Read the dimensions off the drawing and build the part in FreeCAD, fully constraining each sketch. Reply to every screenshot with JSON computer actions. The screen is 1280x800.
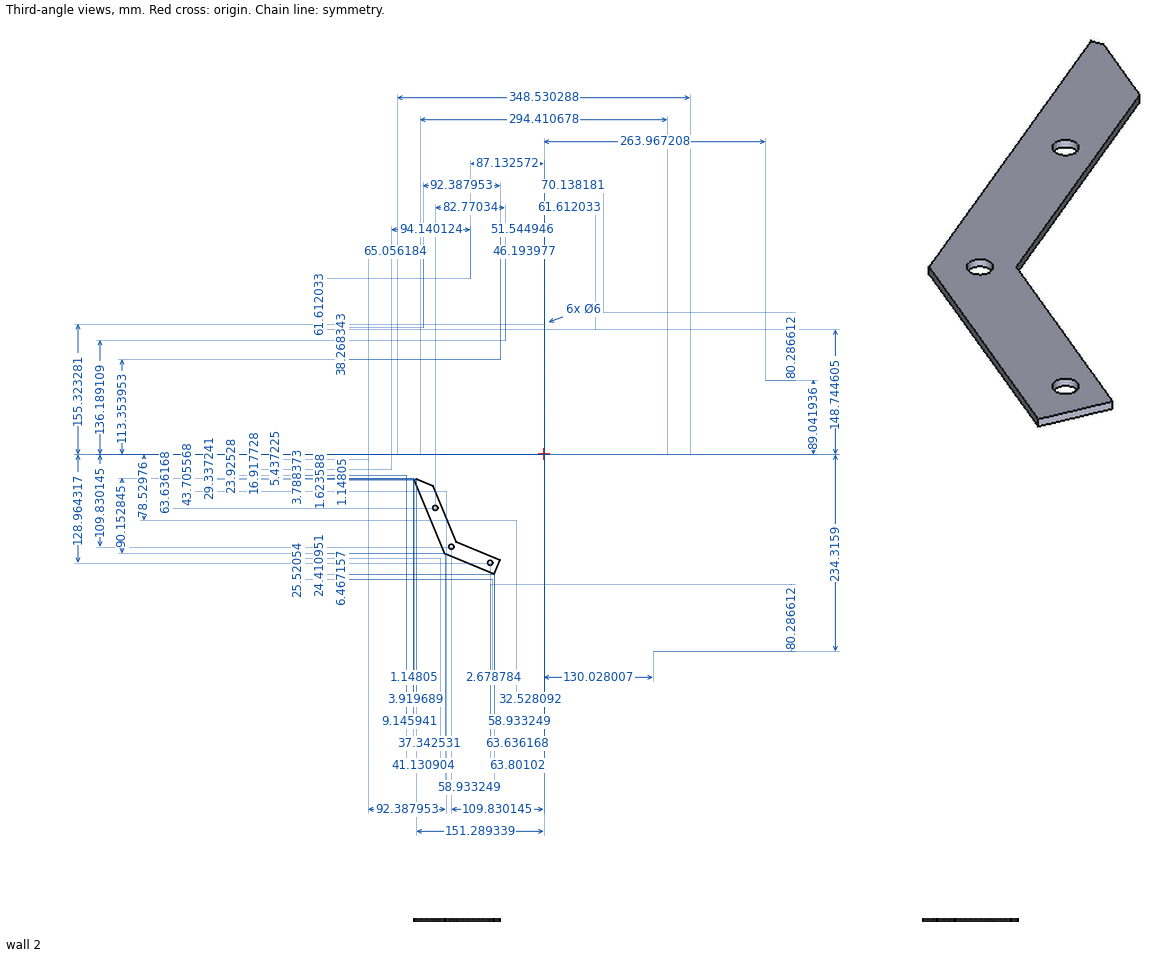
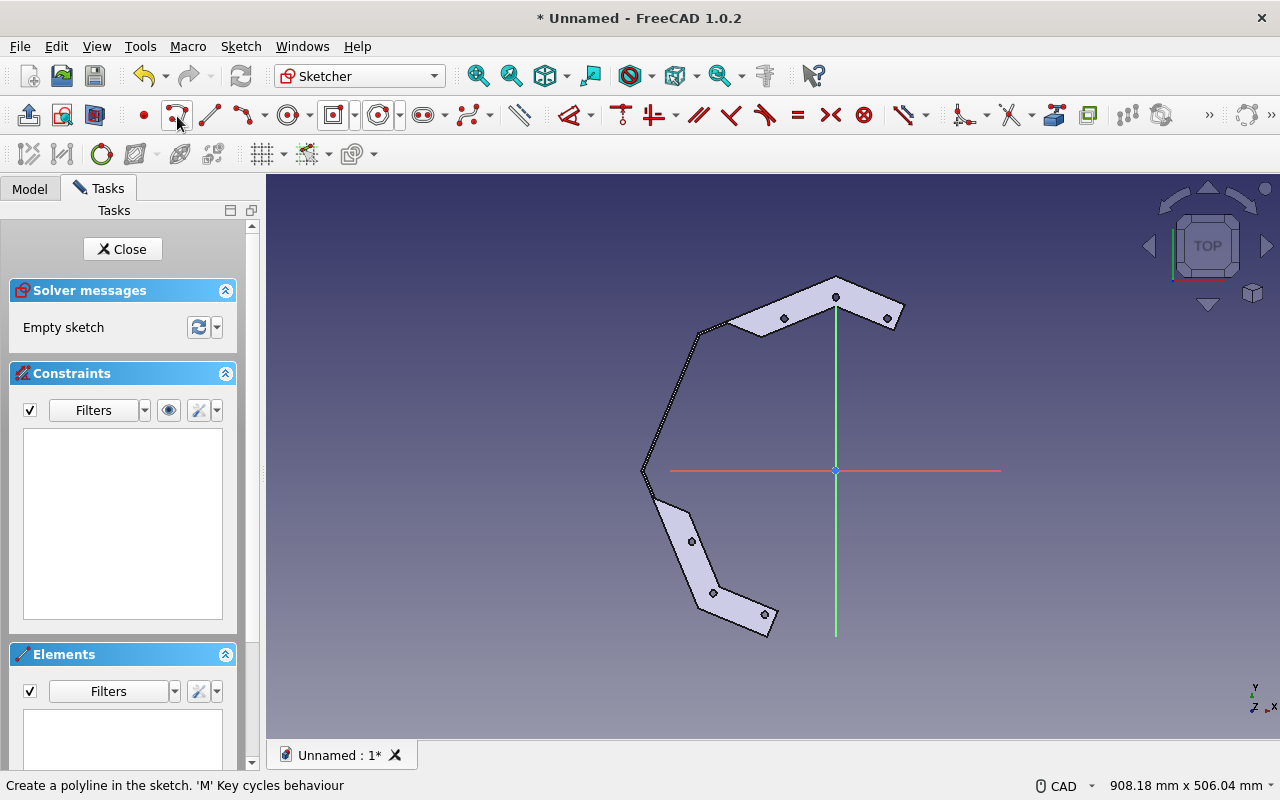
{"action": "left_click", "coordinate": [800, 558]}
{"action": "left_click", "coordinate": [905, 305]}
{"action": "left_click", "coordinate": [739, 236]}
{"action": "left_click", "coordinate": [633, 490]}
{"action": "left_click", "coordinate": [800, 559]}
{"action": "key", "text": "Escape"}
{"action": "key", "text": "Escape"}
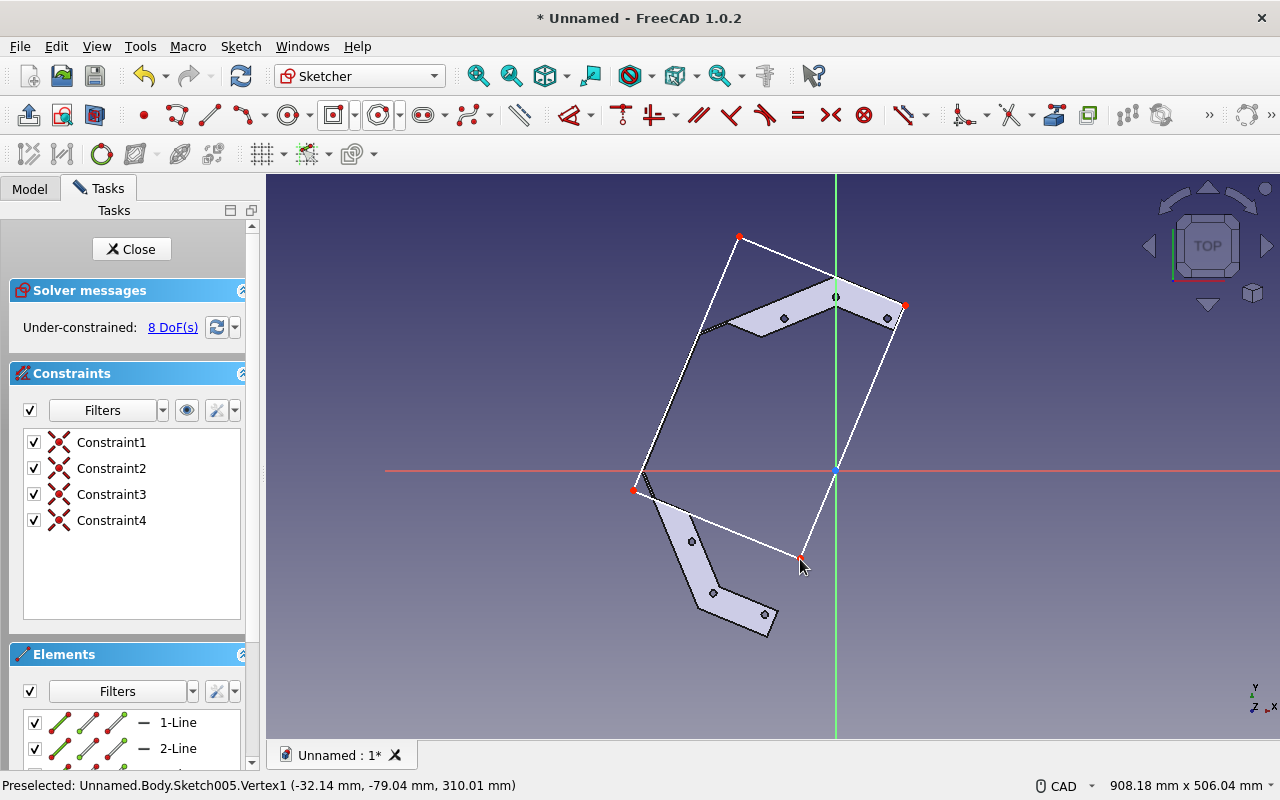
{"action": "left_click", "coordinate": [568, 116]}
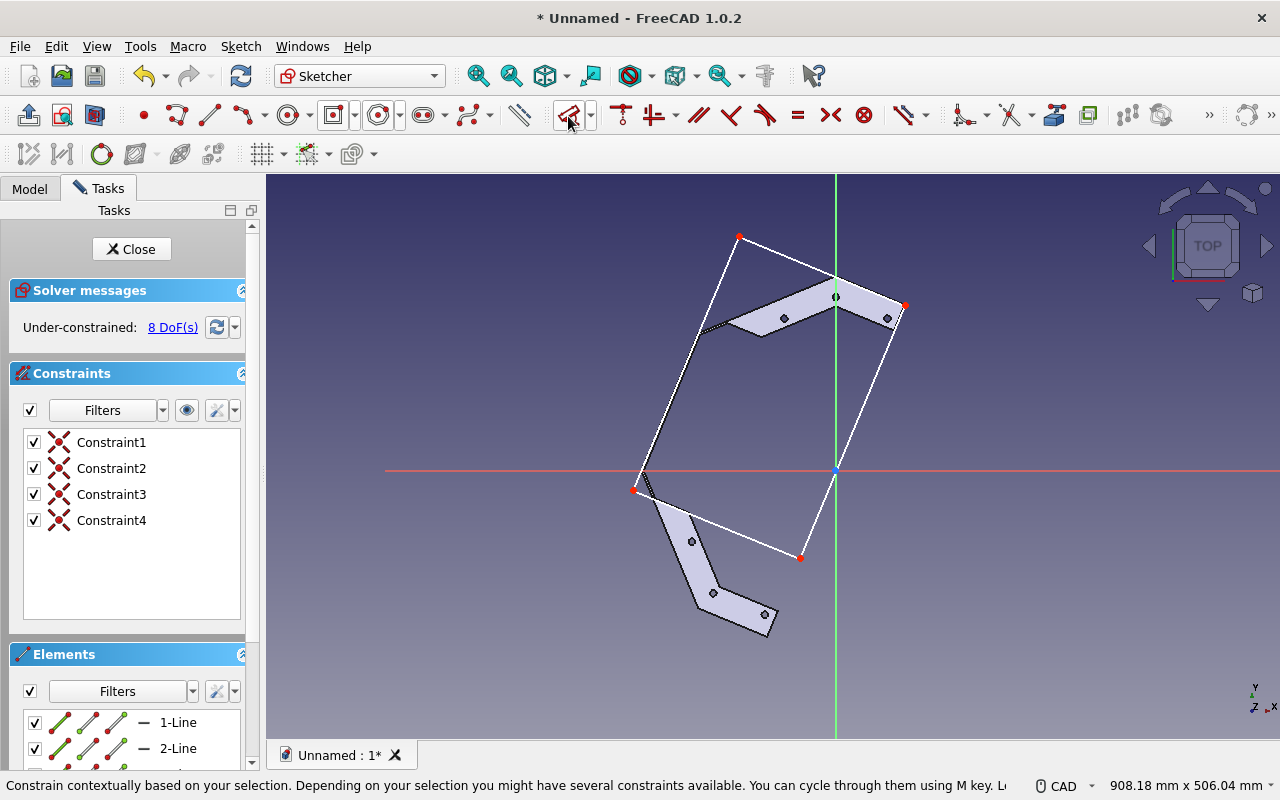
{"action": "left_click", "coordinate": [800, 559]}
{"action": "left_click", "coordinate": [870, 515]}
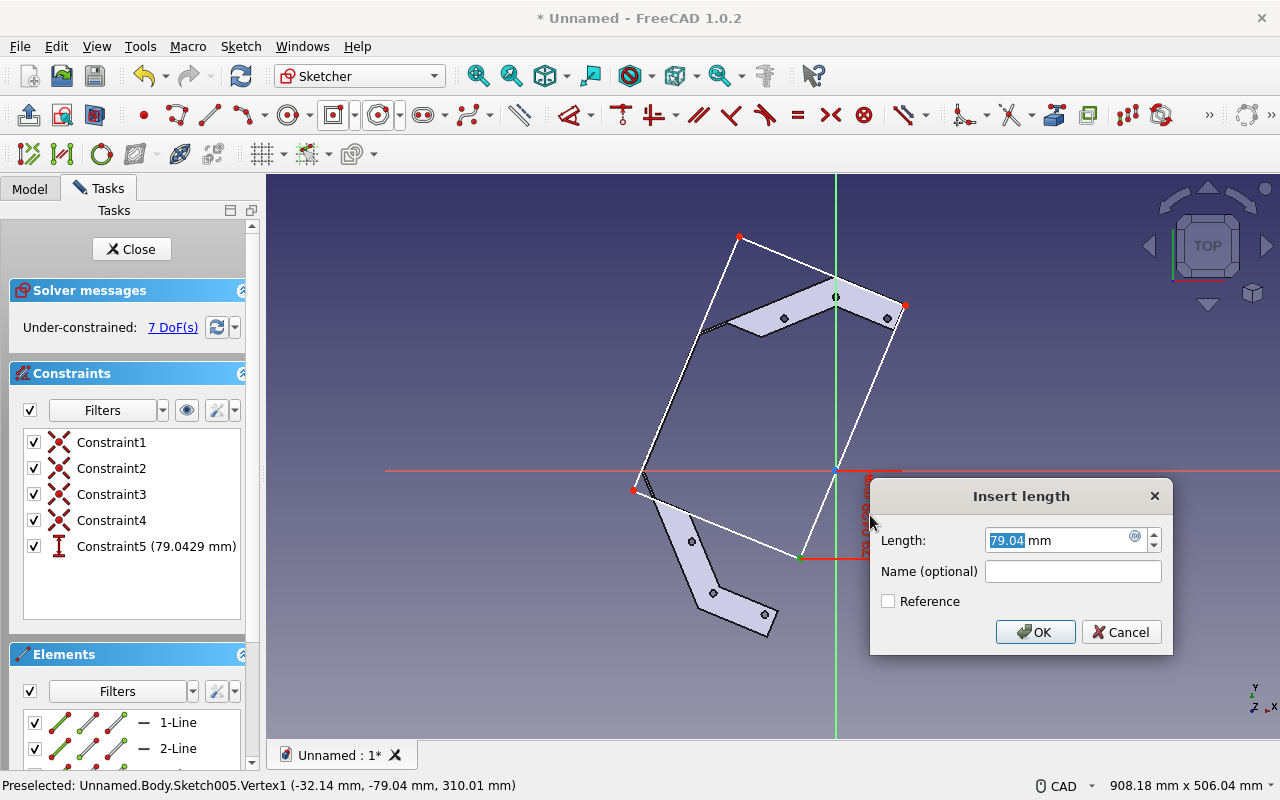
{"action": "type", "text": "78.52976"}
{"action": "key", "text": "Return"}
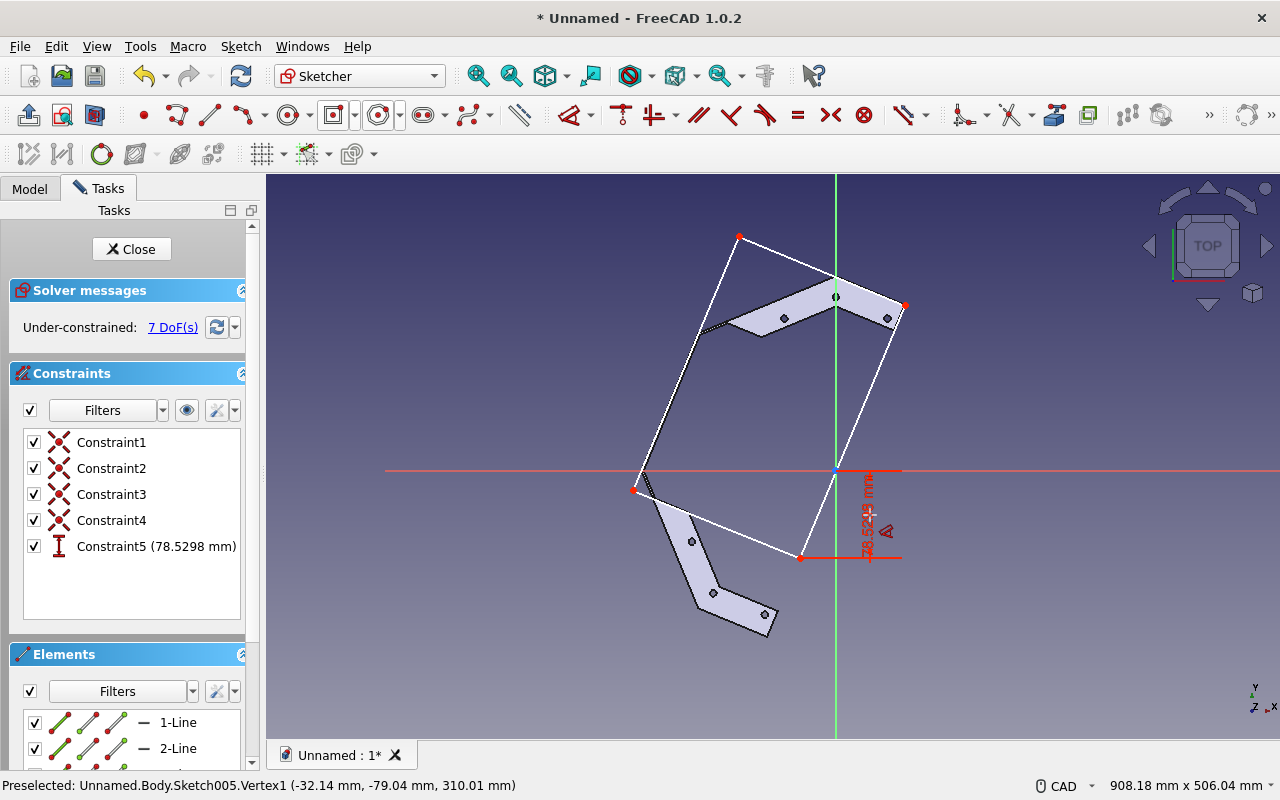
{"action": "left_click", "coordinate": [800, 558]}
{"action": "left_click", "coordinate": [818, 592]}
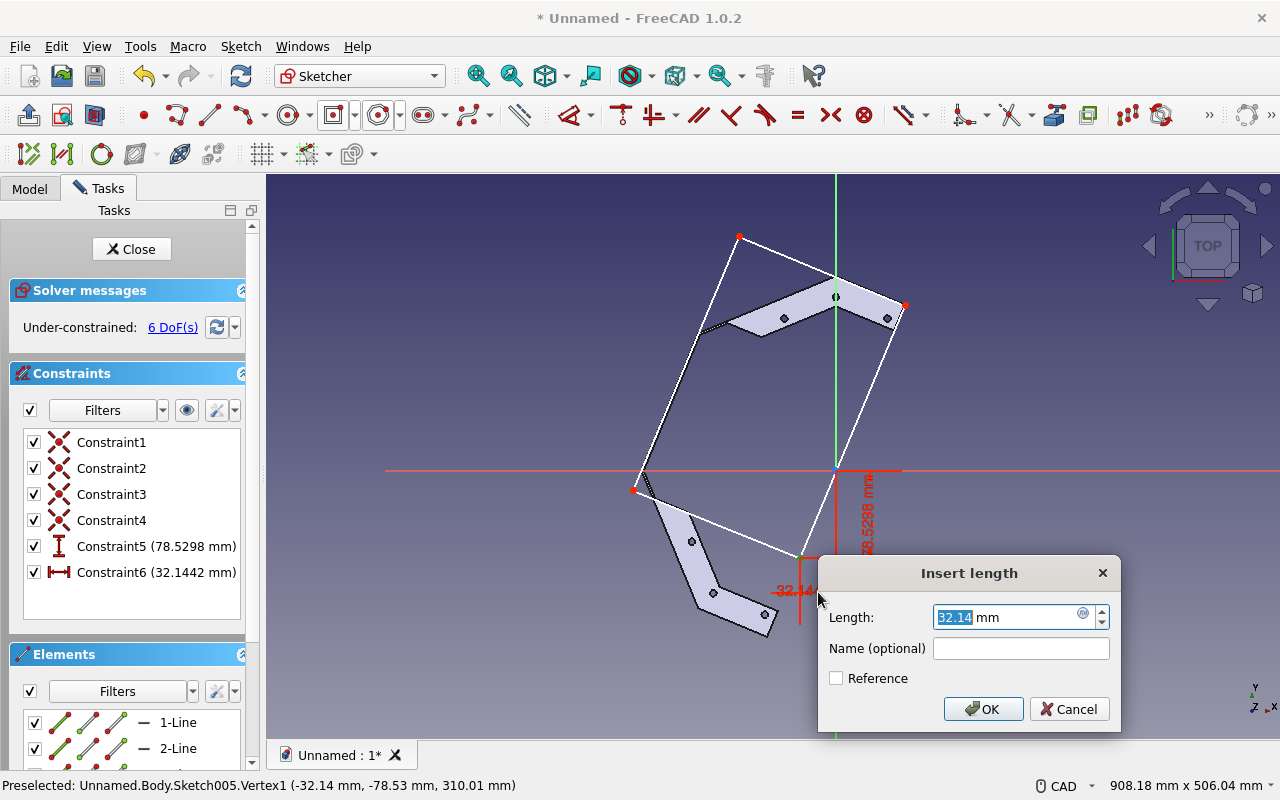
{"action": "type", "text": "32.528092"}
{"action": "key", "text": "Return"}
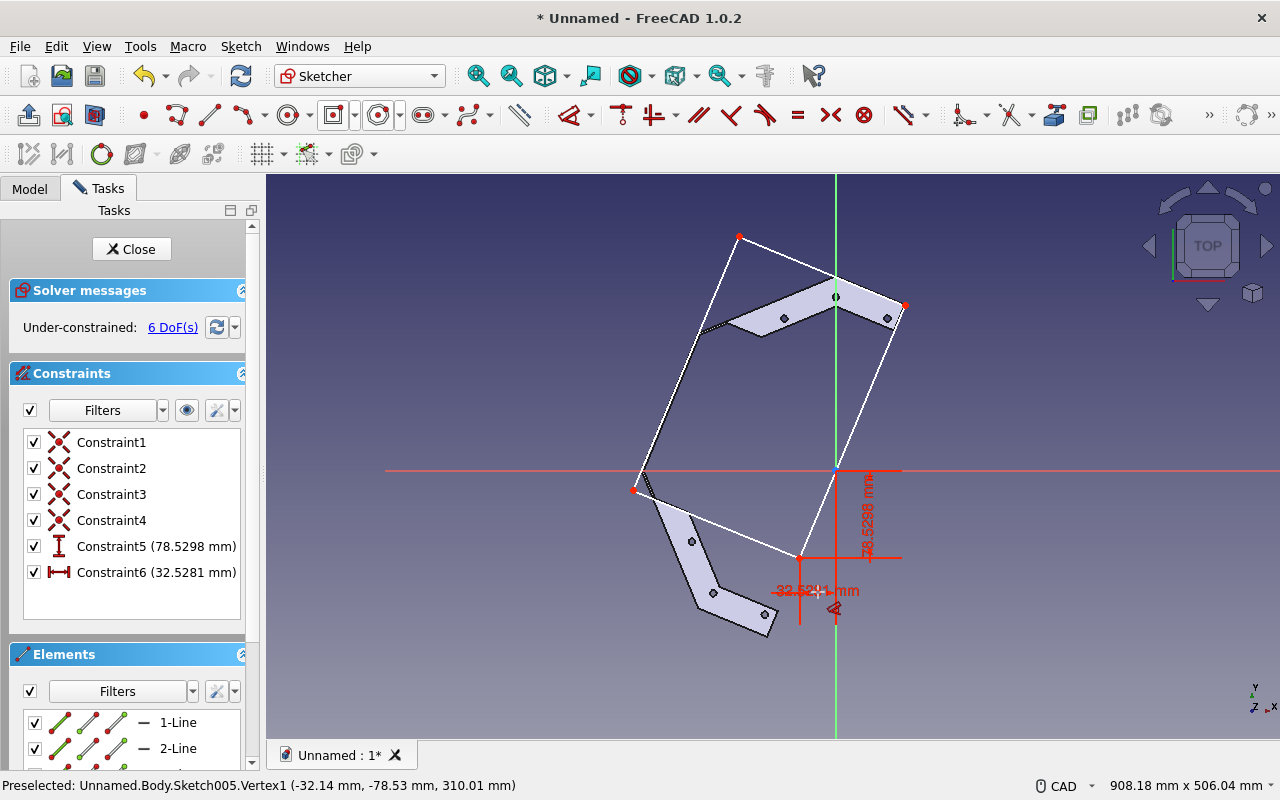
{"action": "left_click", "coordinate": [905, 306]}
{"action": "left_click", "coordinate": [870, 272]}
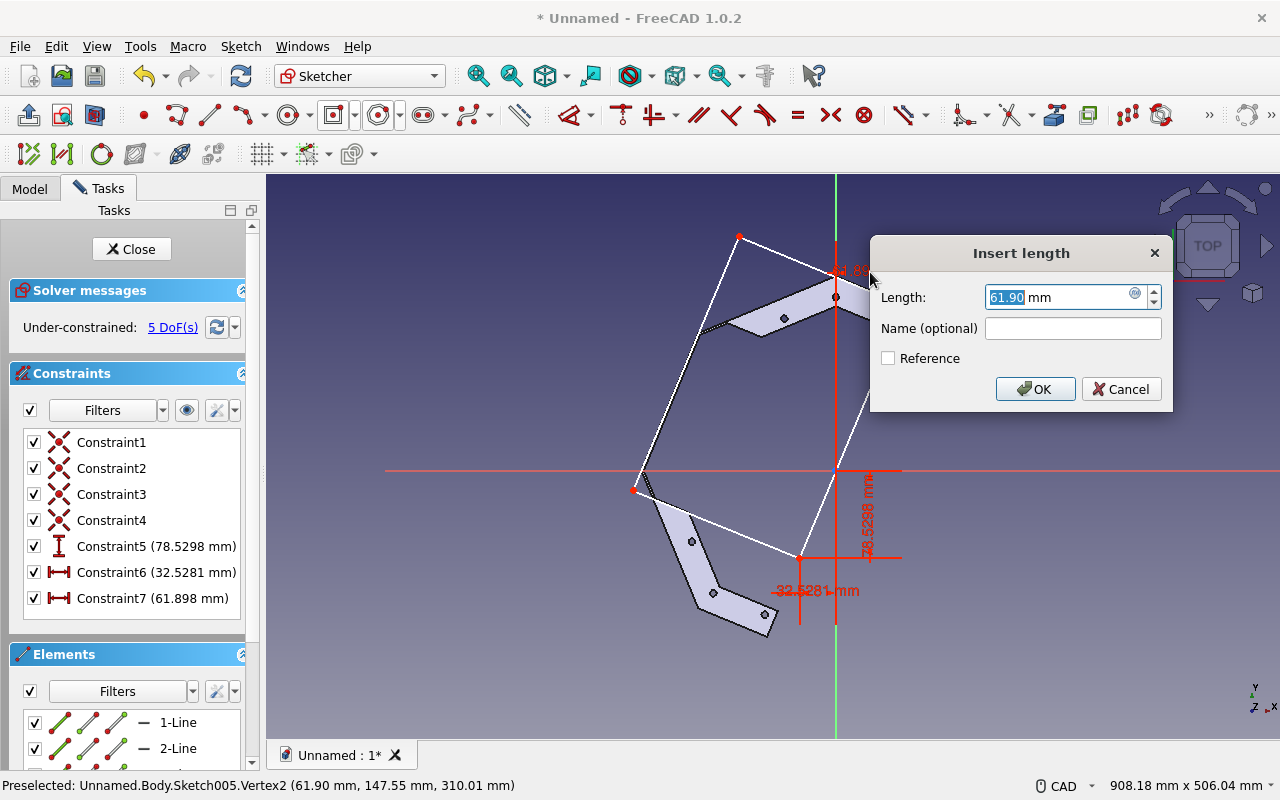
{"action": "type", "text": "61.612033"}
{"action": "key", "text": "Return"}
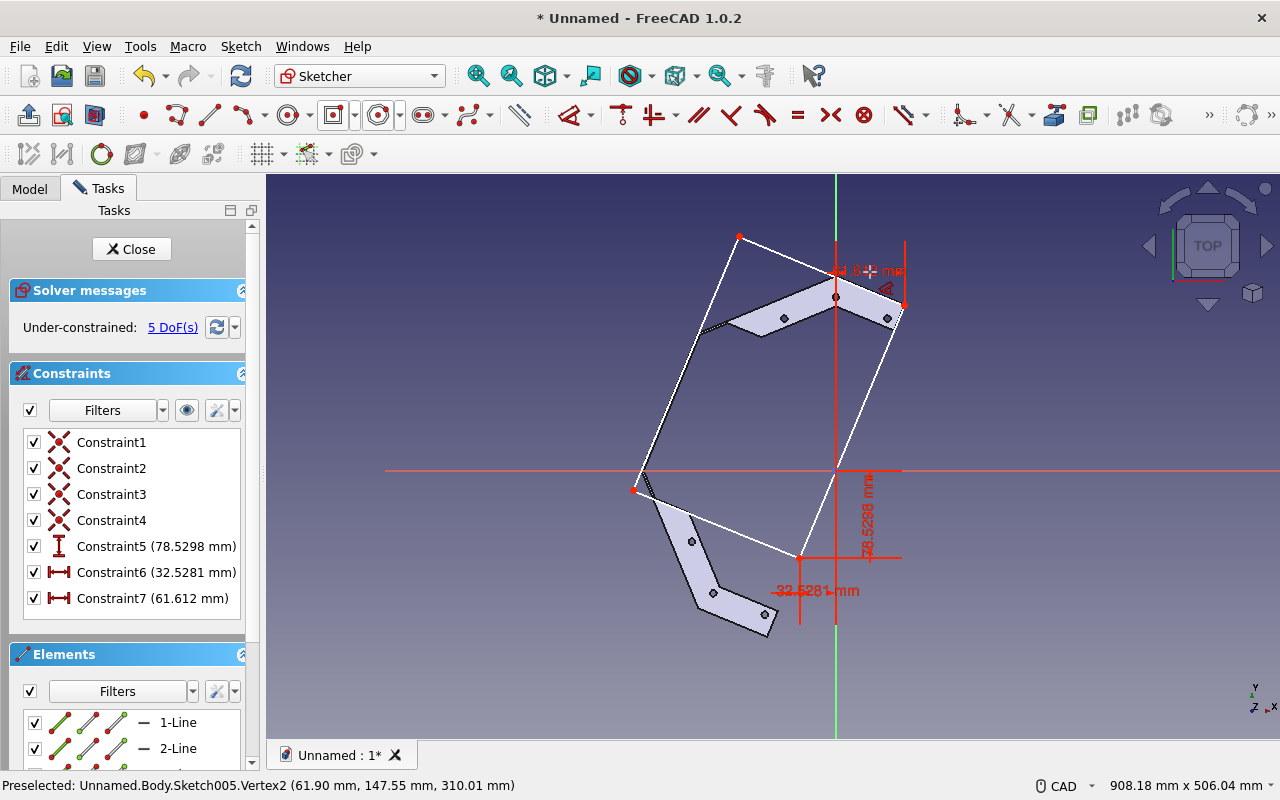
{"action": "left_click", "coordinate": [739, 237]}
{"action": "left_click", "coordinate": [787, 203]}